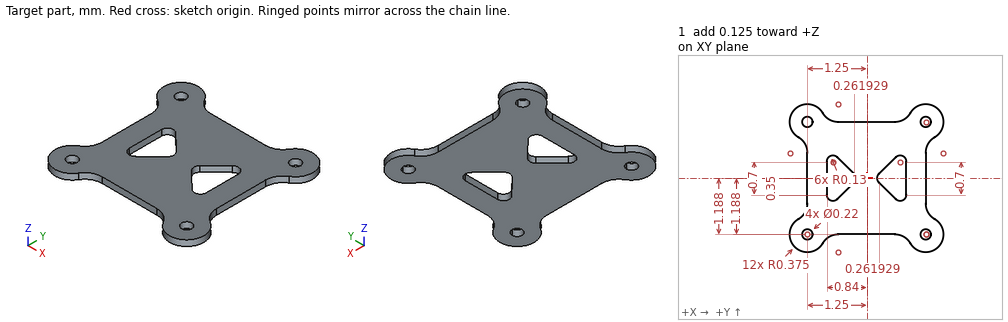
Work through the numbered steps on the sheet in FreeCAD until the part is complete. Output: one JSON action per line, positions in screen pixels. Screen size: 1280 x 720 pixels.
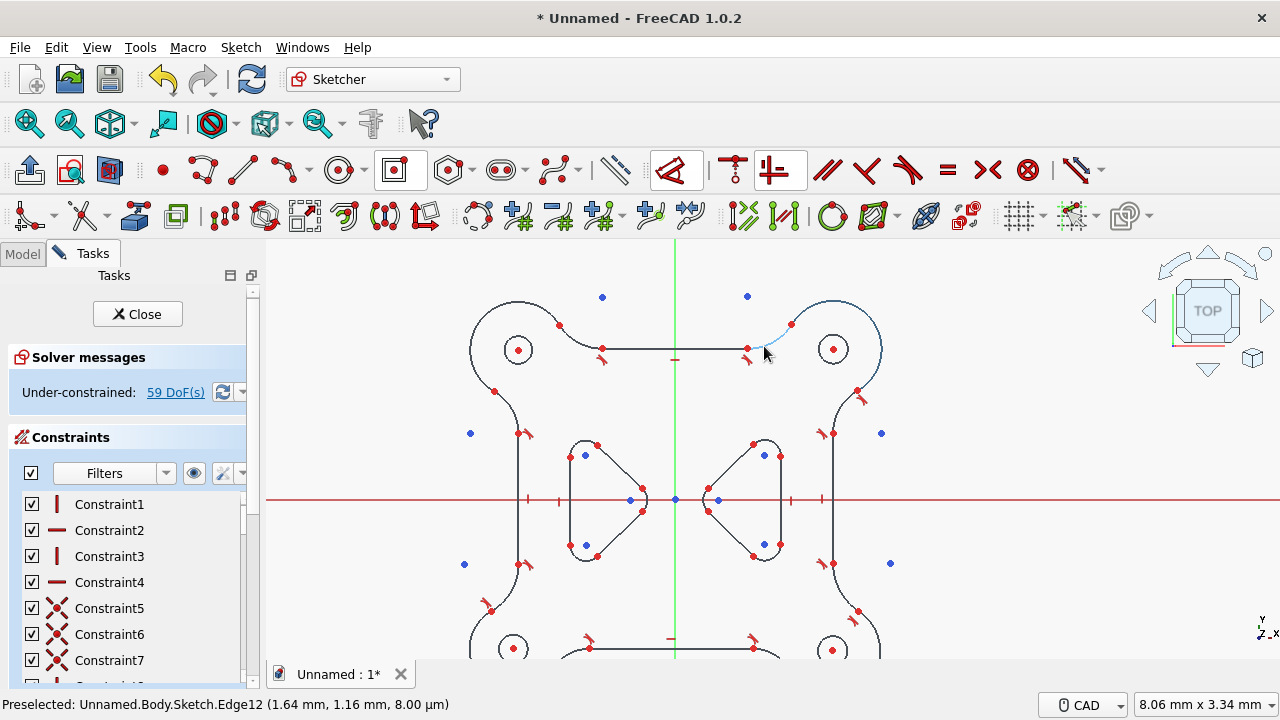
{"action": "left_click", "coordinate": [763, 346]}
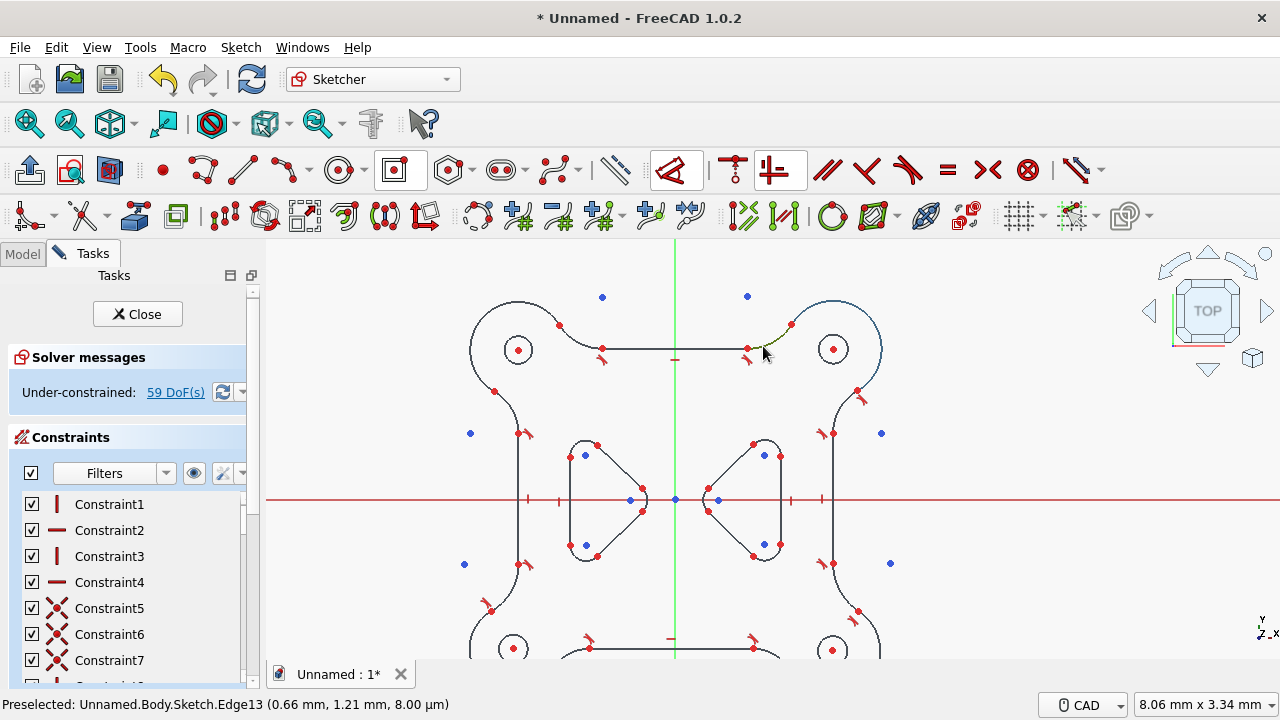
{"action": "left_click", "coordinate": [908, 170]}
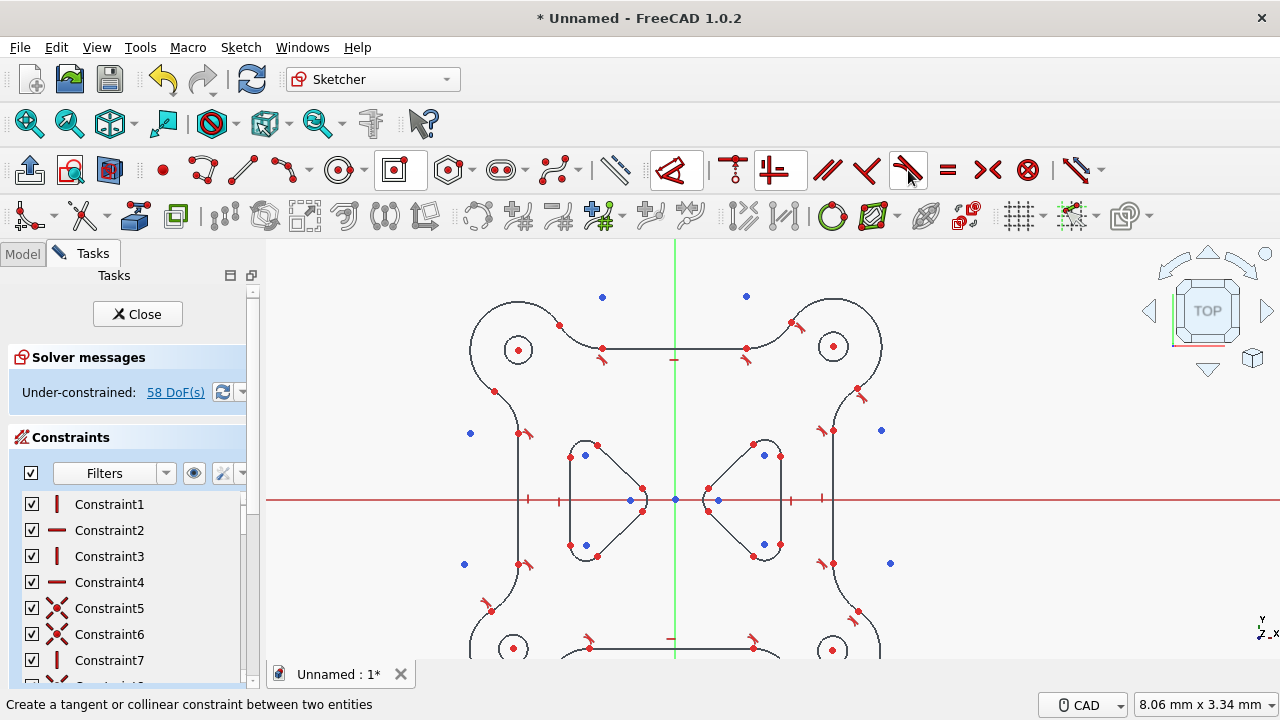
{"action": "left_click", "coordinate": [570, 337]}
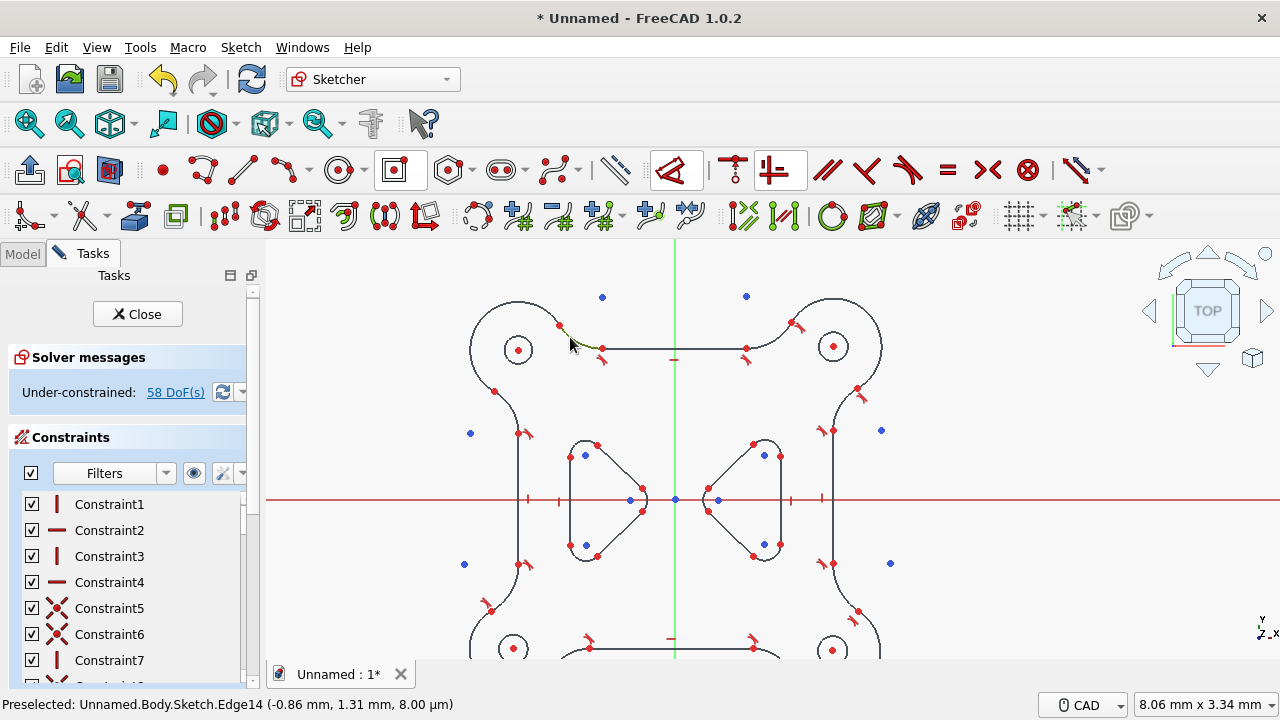
{"action": "left_click", "coordinate": [516, 302]}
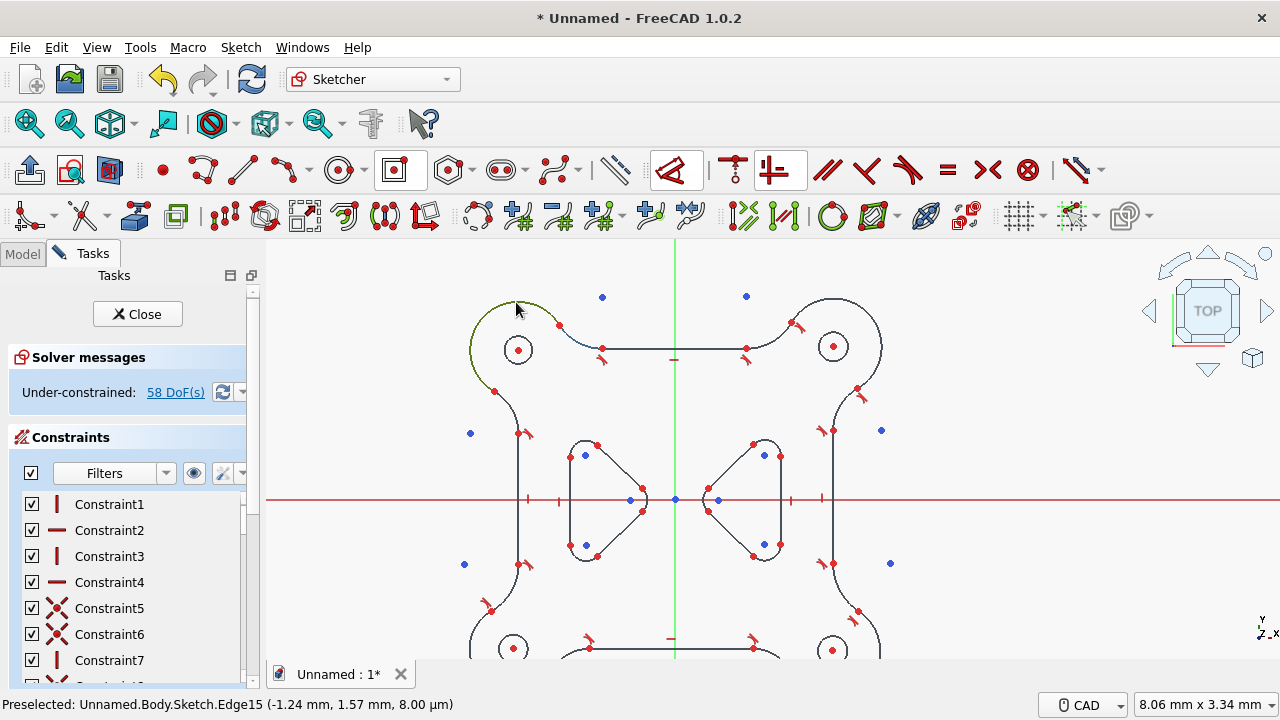
{"action": "left_click", "coordinate": [908, 170]}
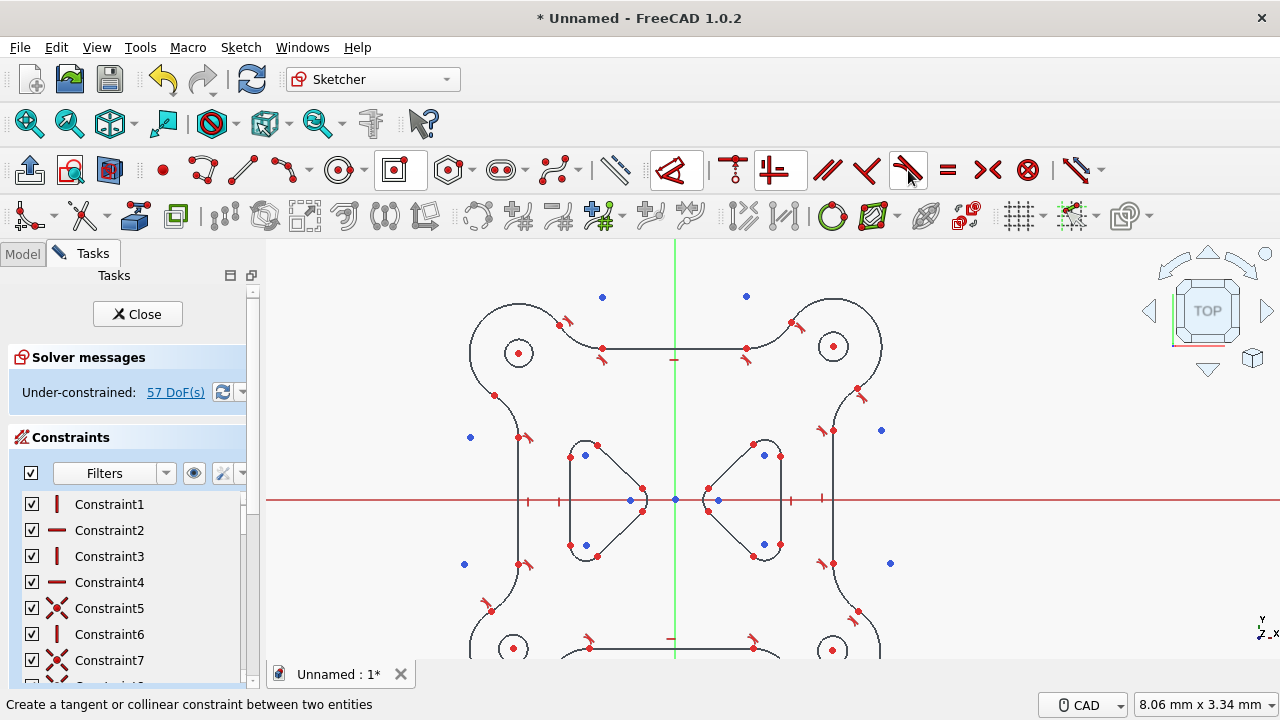
{"action": "left_click", "coordinate": [514, 304]}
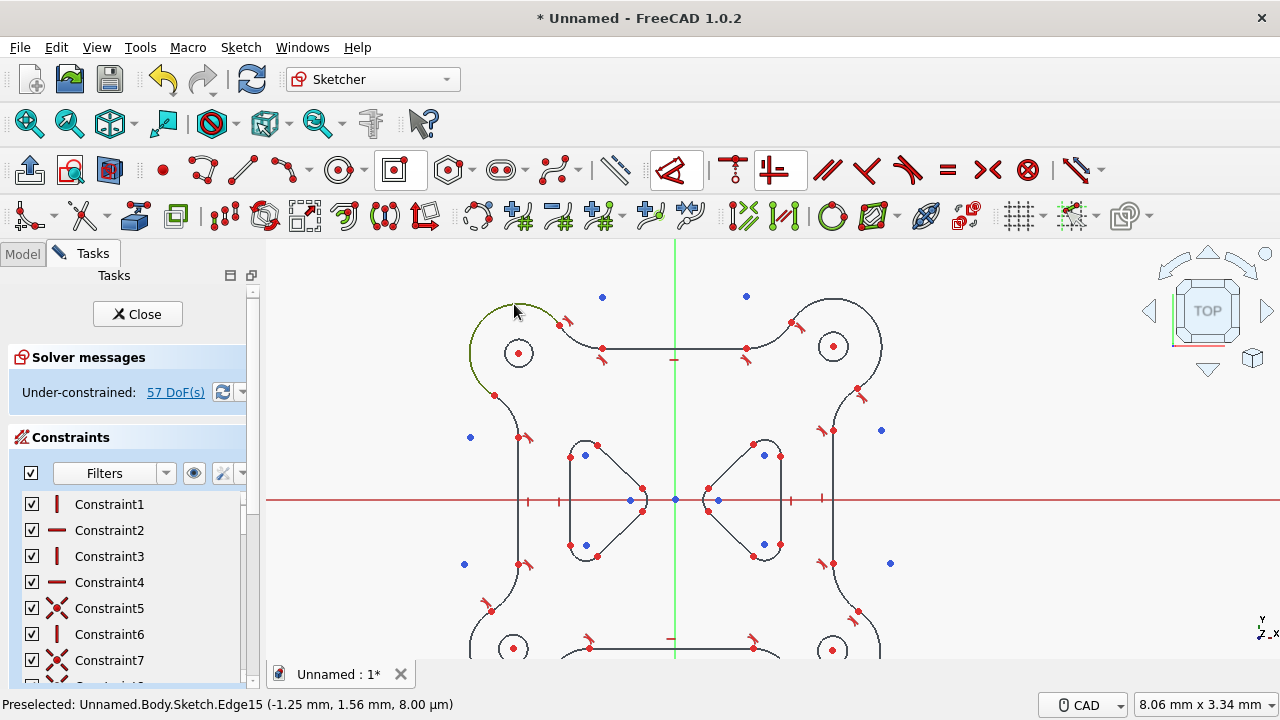
{"action": "left_click", "coordinate": [516, 423]}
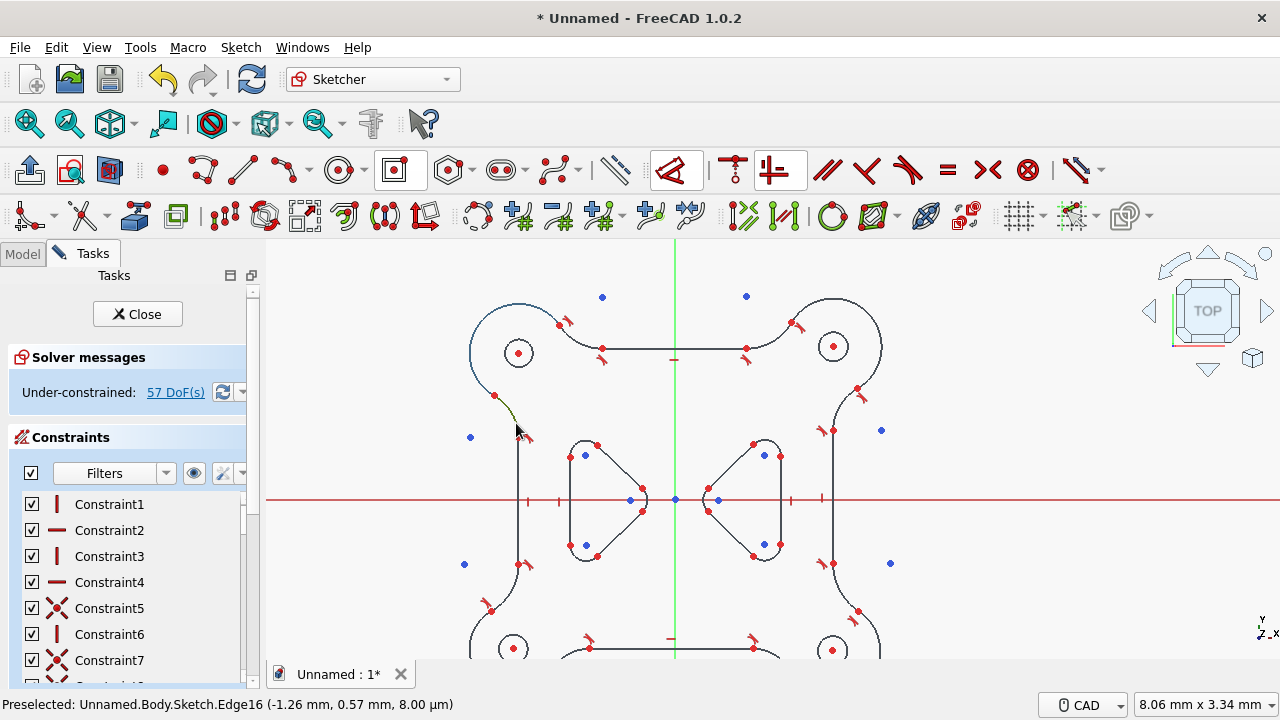
{"action": "left_click", "coordinate": [908, 170]}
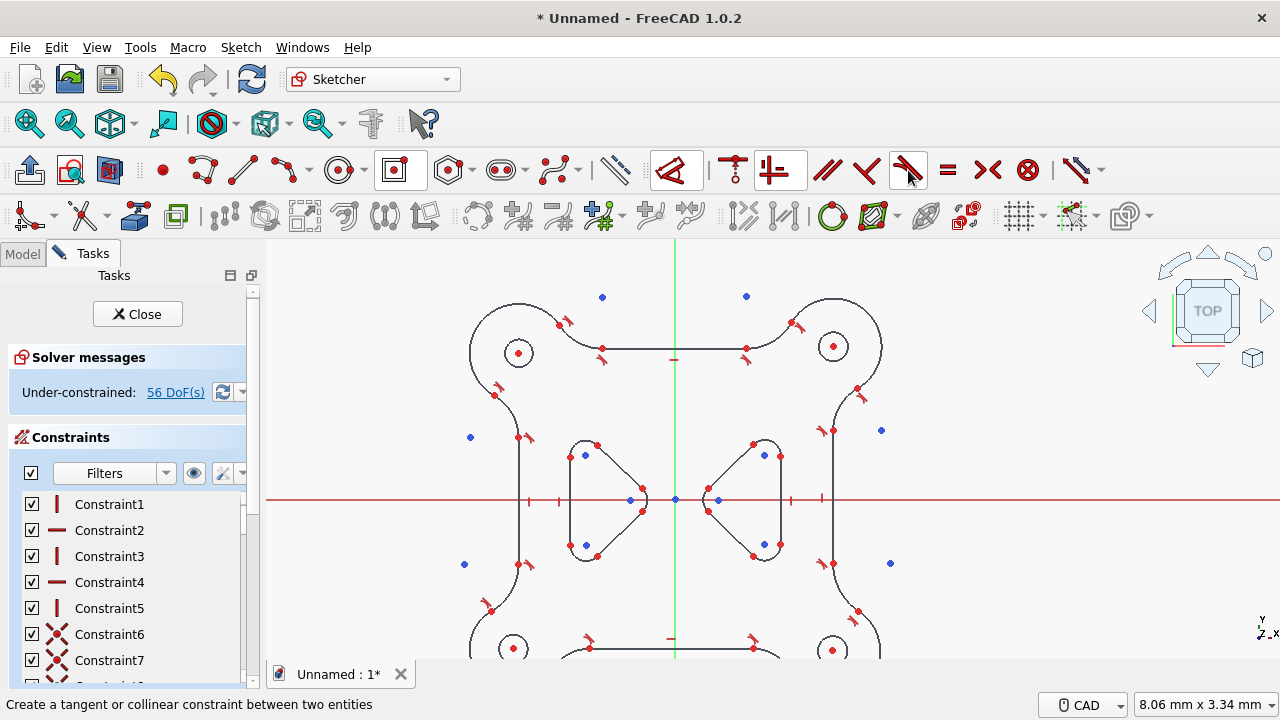
{"action": "left_click", "coordinate": [570, 519]}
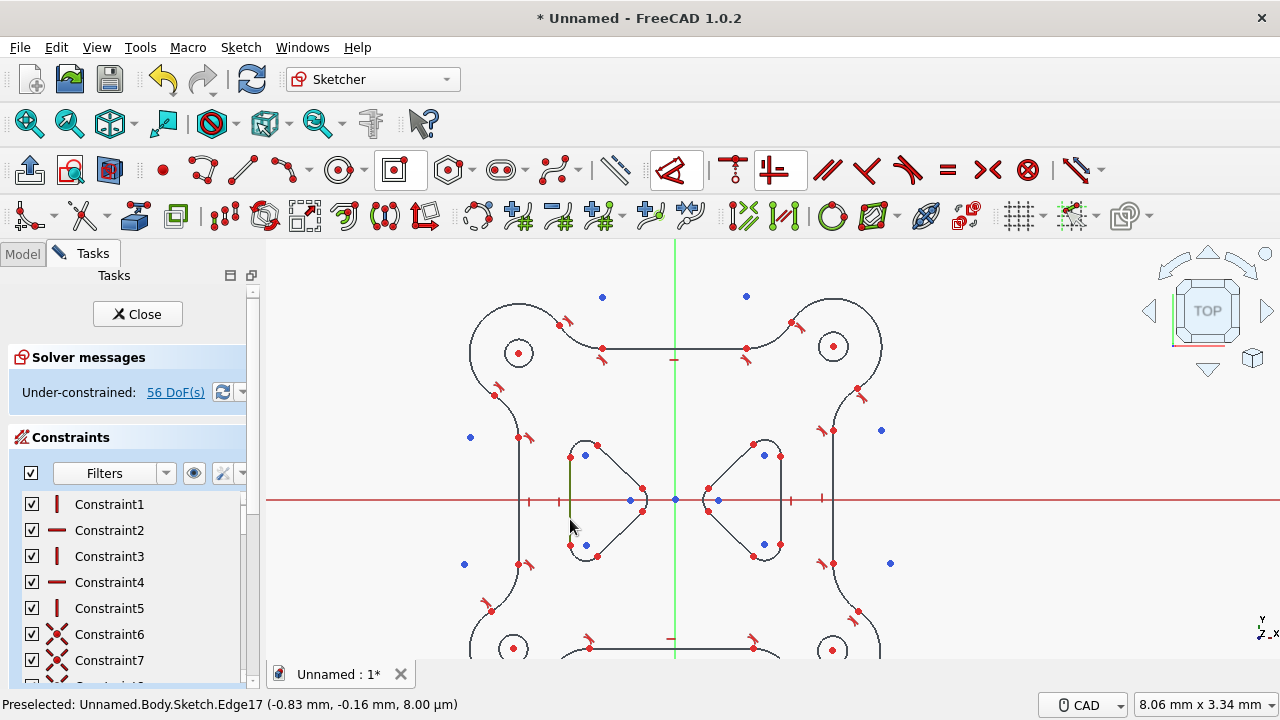
{"action": "left_click", "coordinate": [587, 441]}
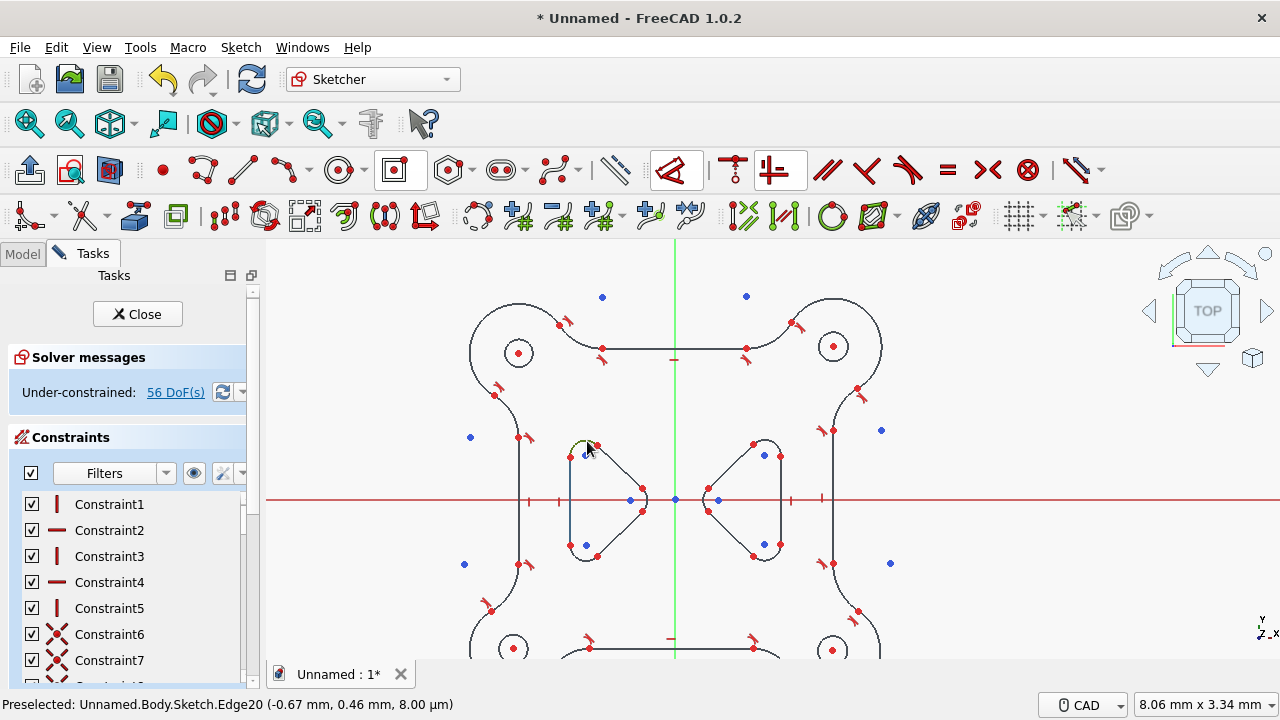
{"action": "left_click", "coordinate": [908, 170]}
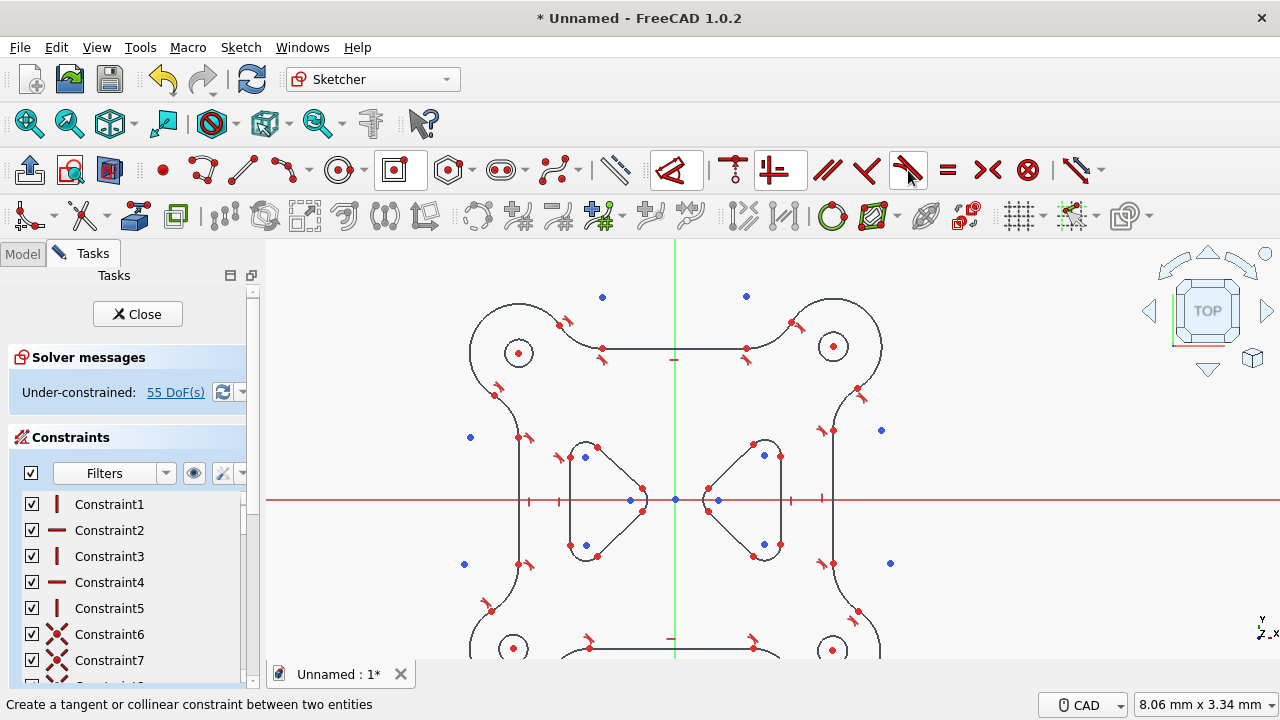
{"action": "left_click", "coordinate": [570, 519]}